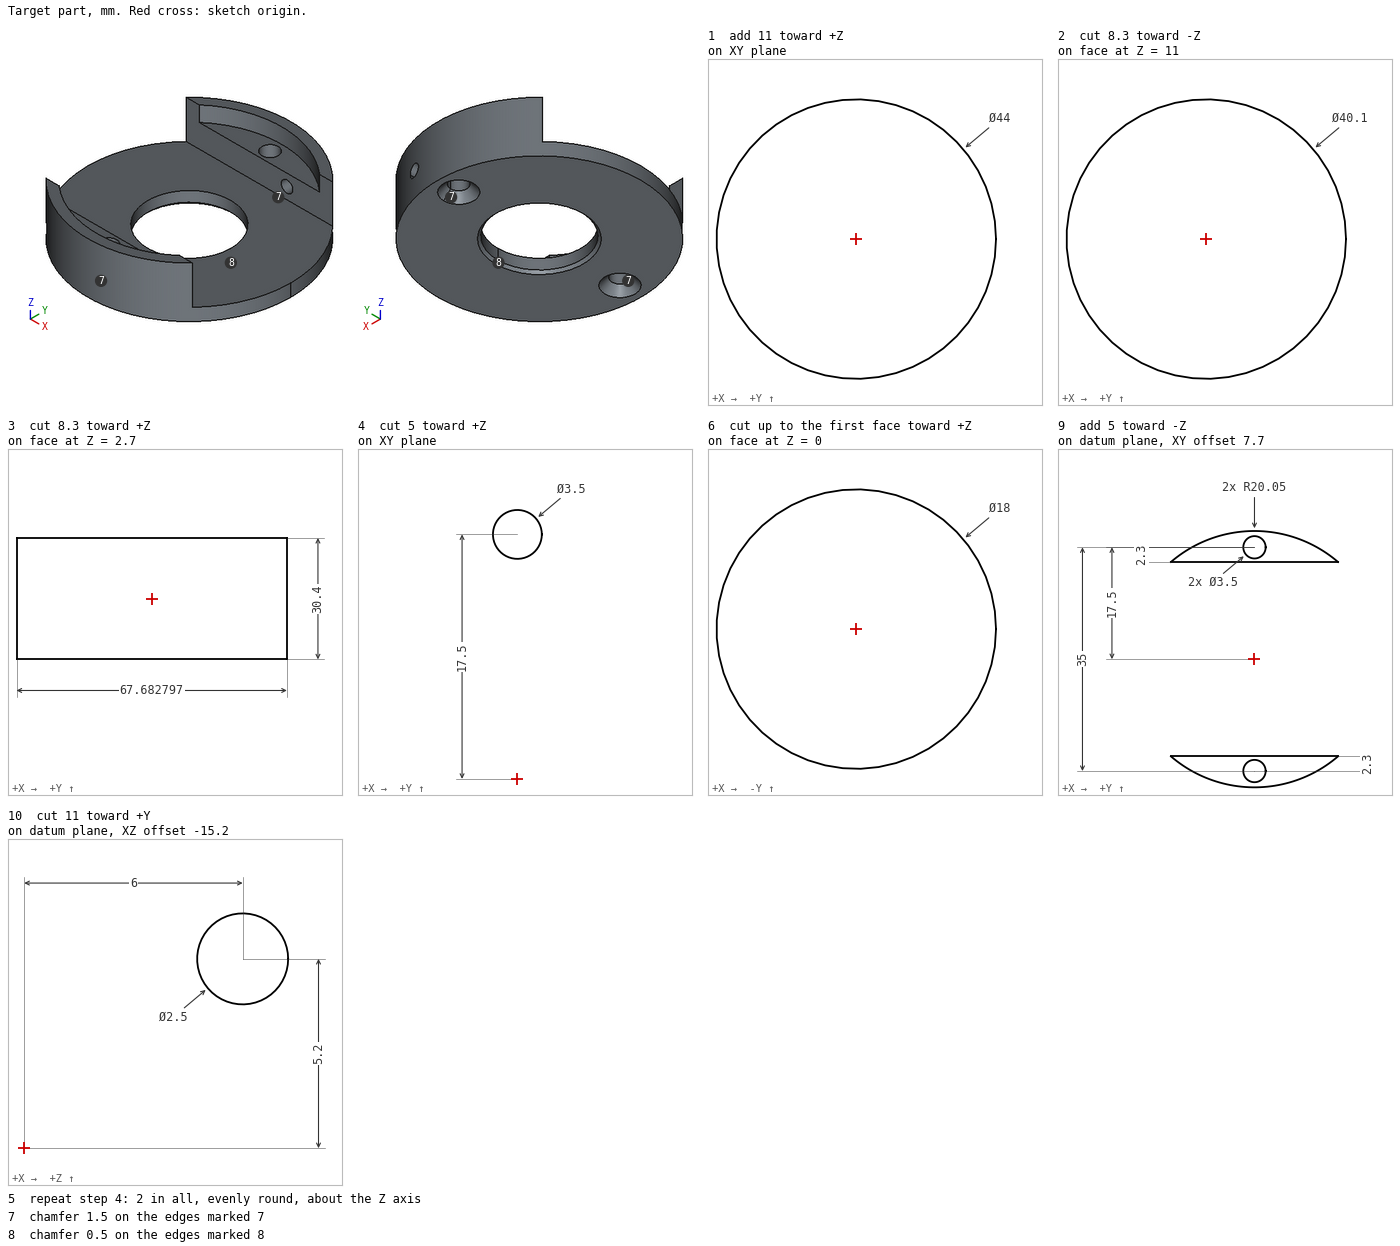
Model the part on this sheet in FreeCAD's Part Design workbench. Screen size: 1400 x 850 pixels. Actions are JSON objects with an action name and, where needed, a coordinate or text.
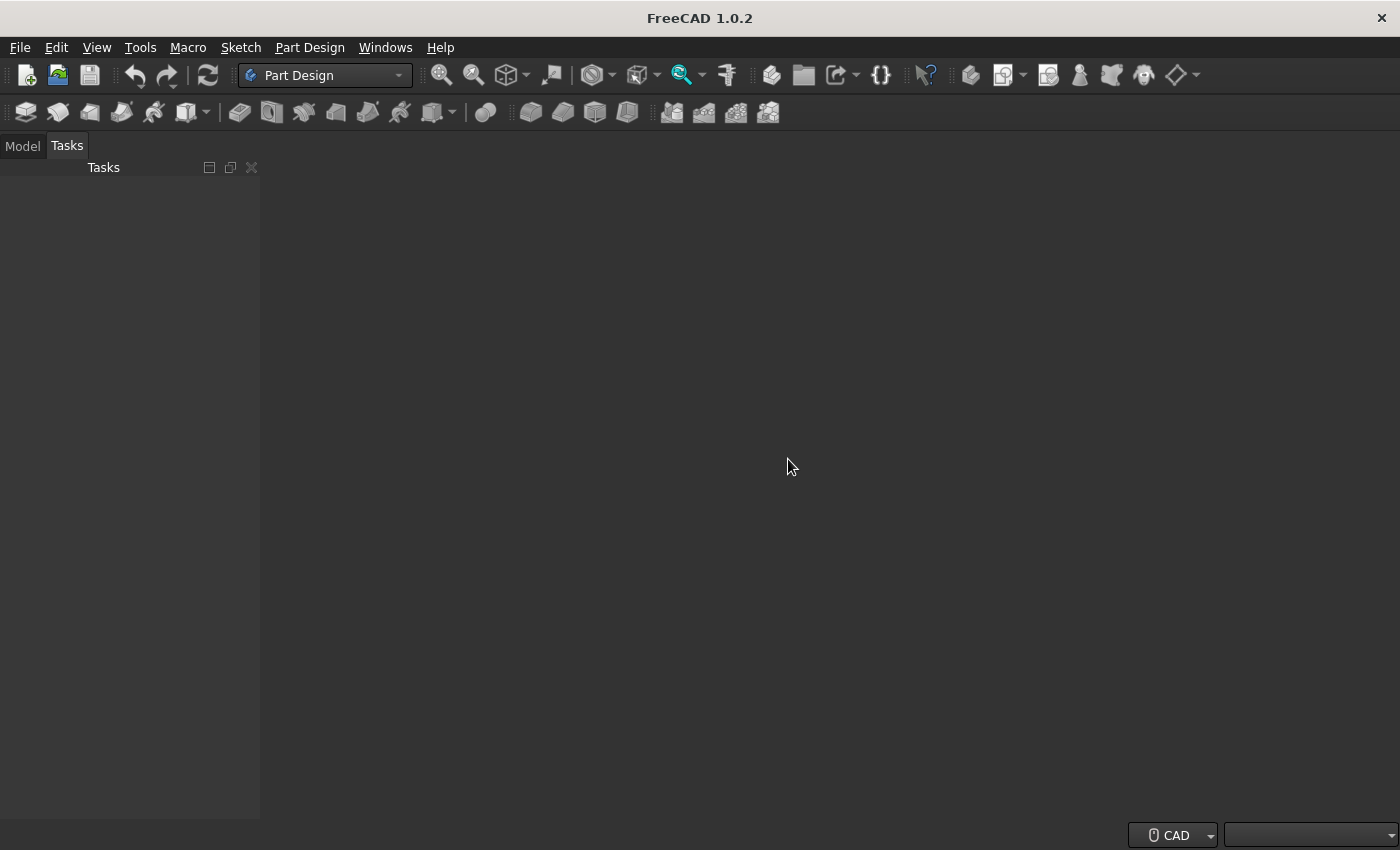
{"action": "left_click", "coordinate": [26, 76]}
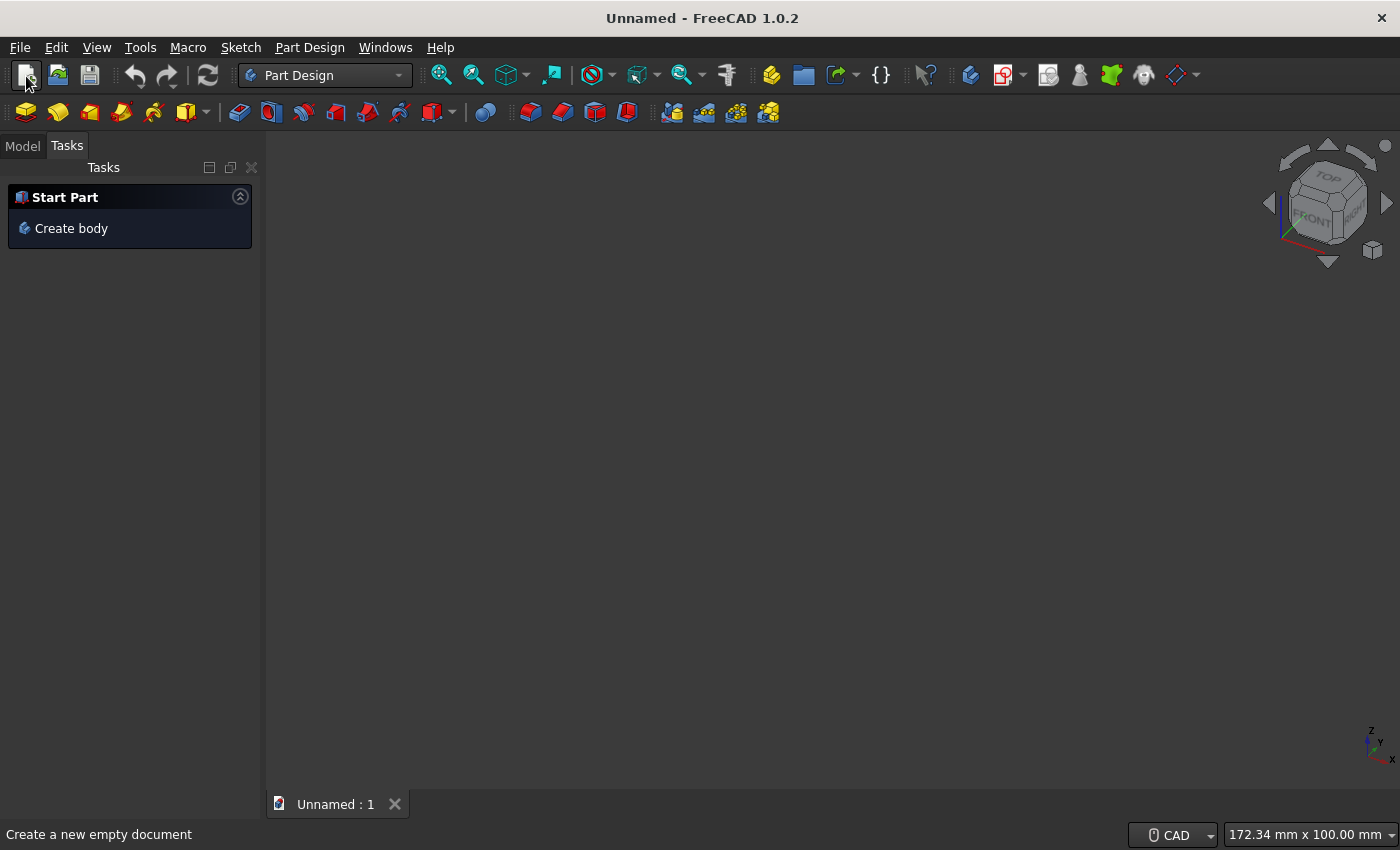
{"action": "left_click", "coordinate": [1004, 76]}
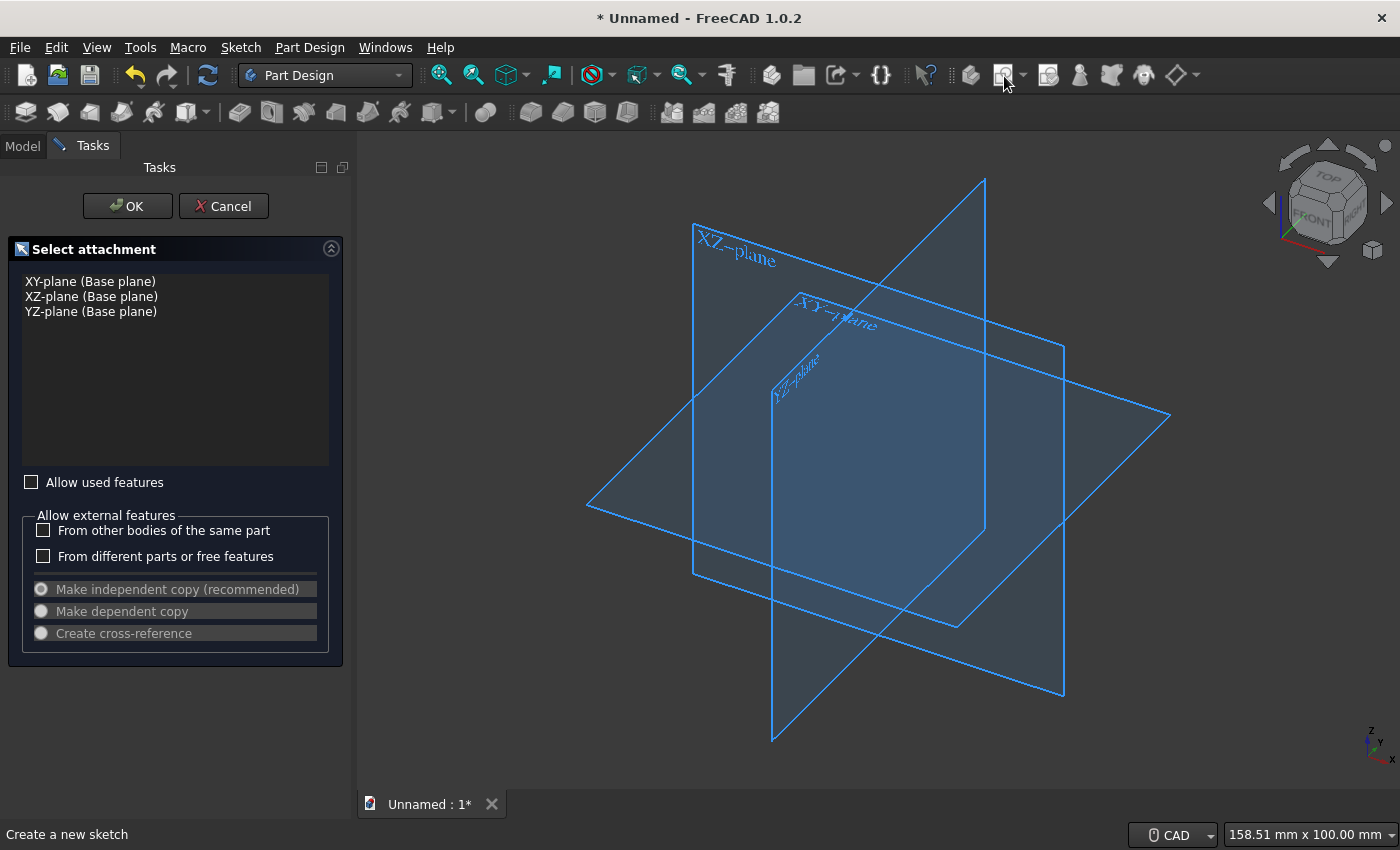
{"action": "left_click", "coordinate": [82, 282]}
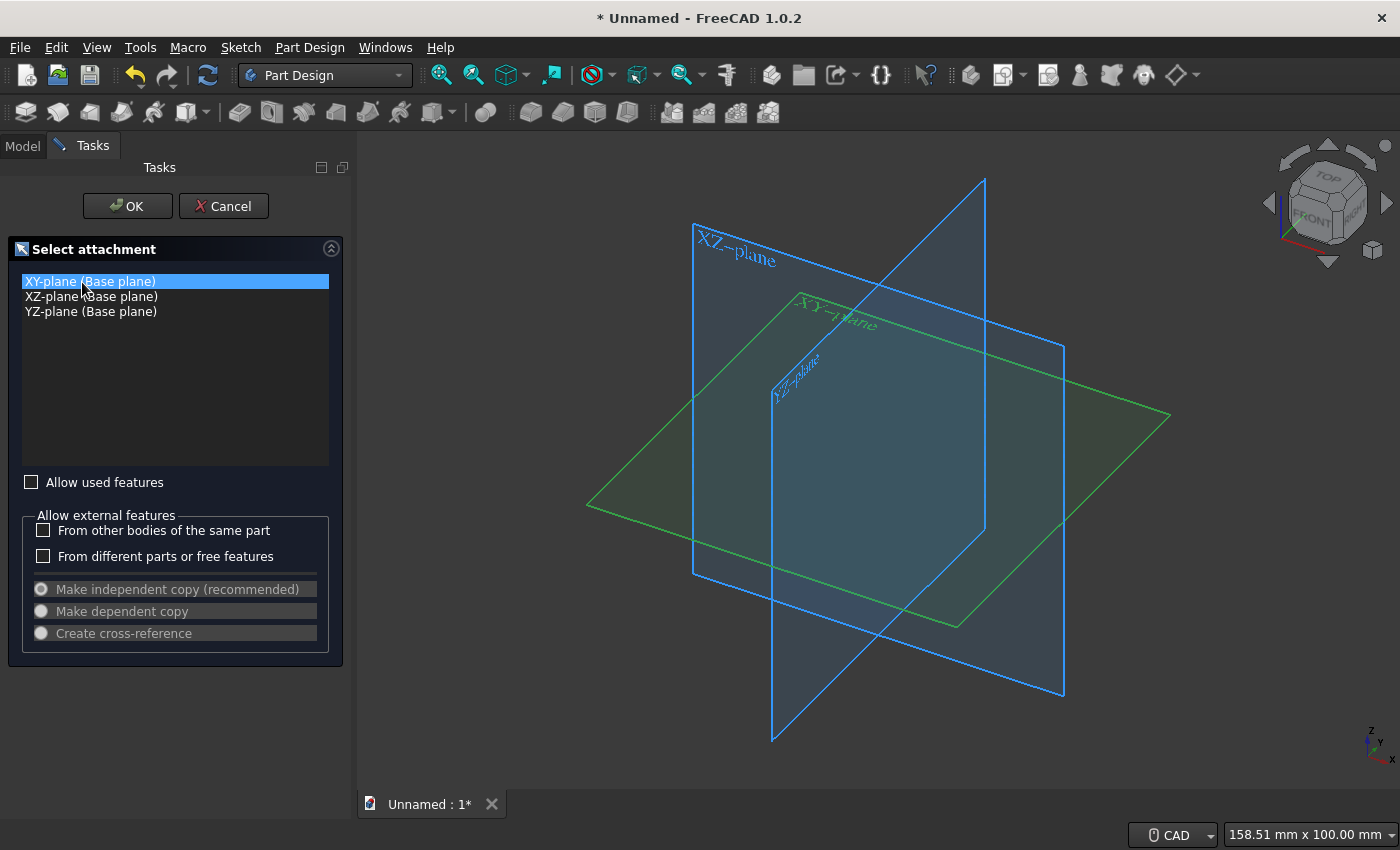
{"action": "left_click", "coordinate": [128, 206]}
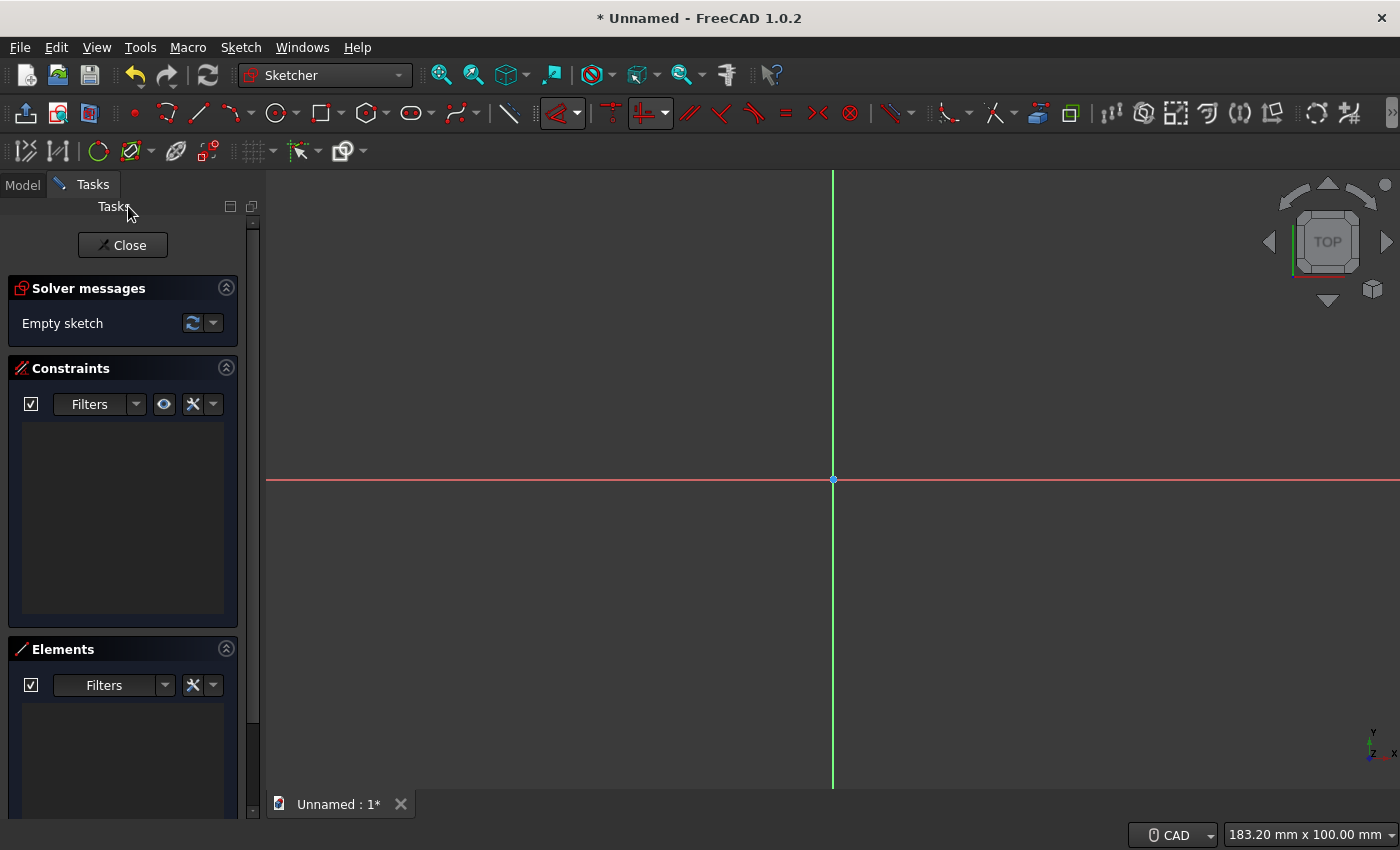
{"action": "scroll", "coordinate": [972, 480], "scroll_direction": "up", "scroll_amount": 2}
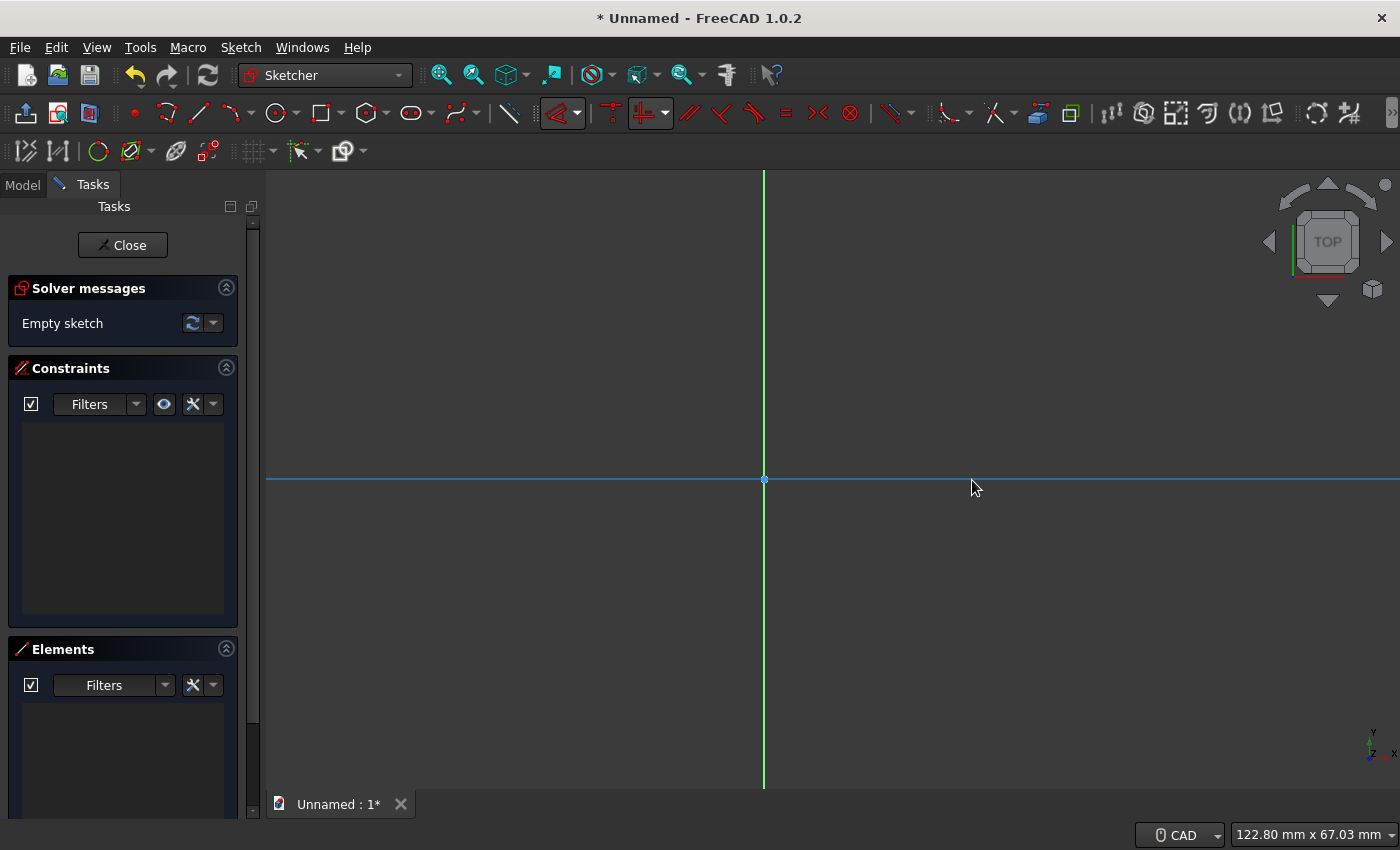
{"action": "key", "text": "g c"}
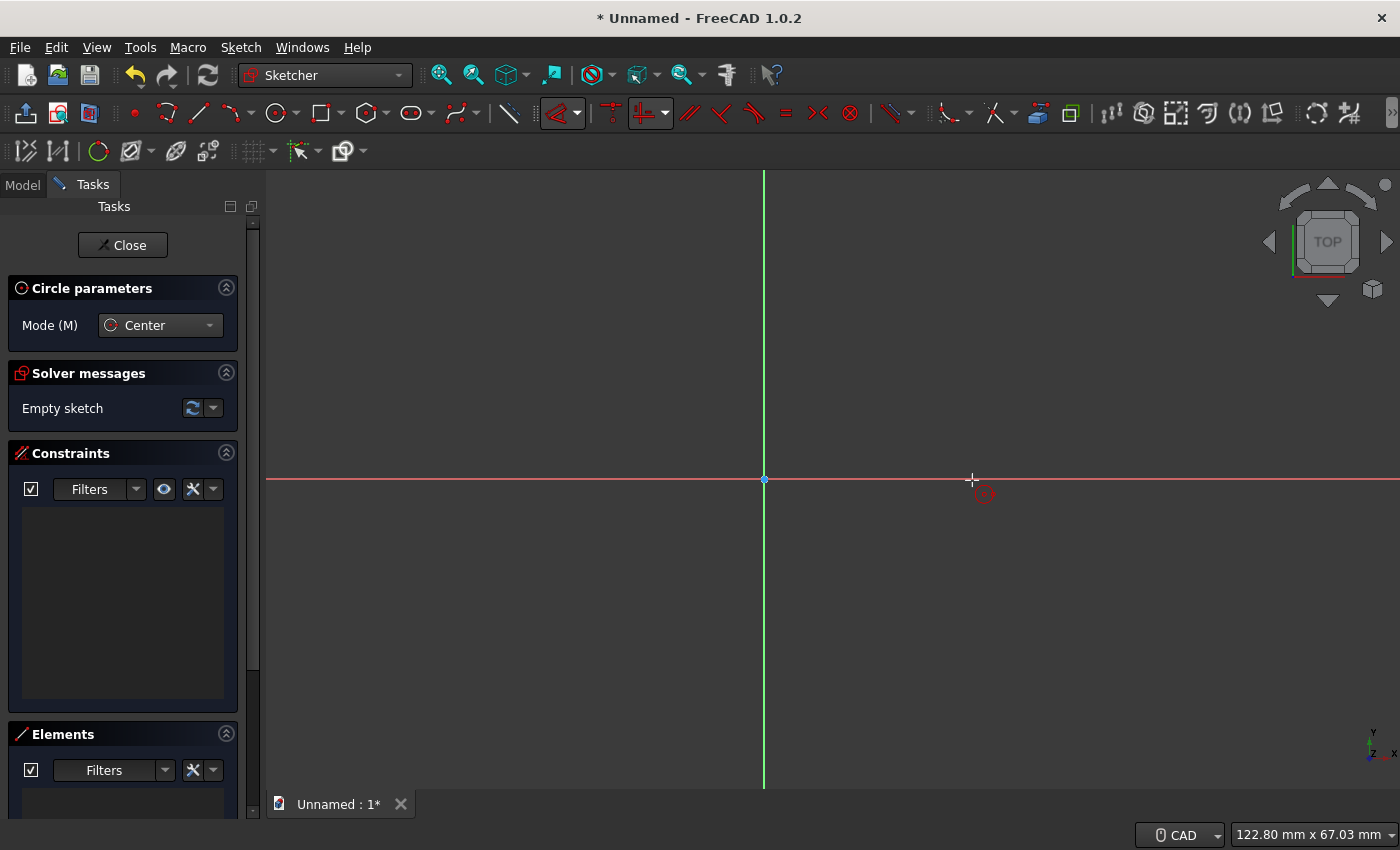
{"action": "left_click", "coordinate": [764, 479]}
{"action": "left_click", "coordinate": [908, 335]}
{"action": "key", "text": "Escape"}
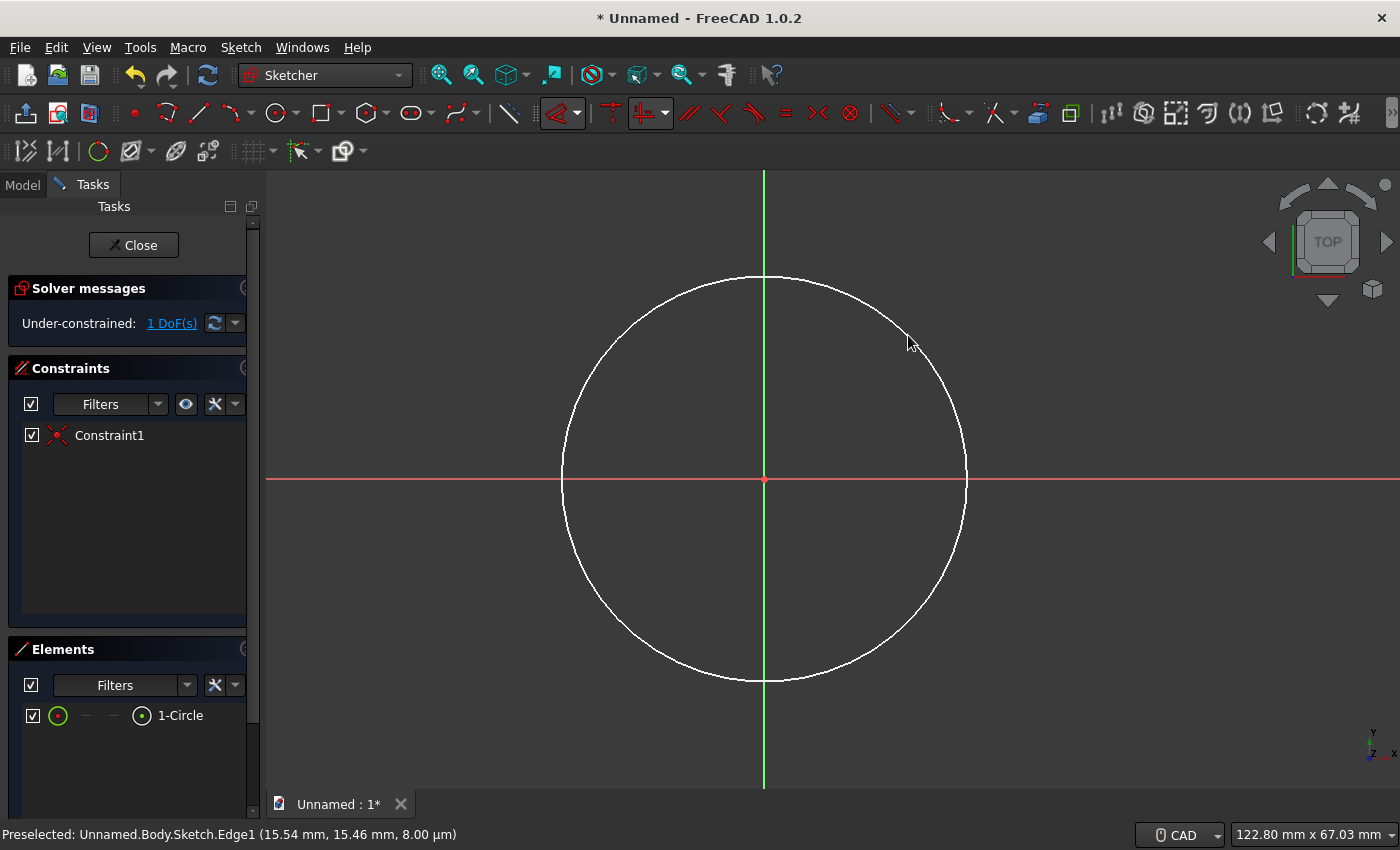
{"action": "key", "text": "d"}